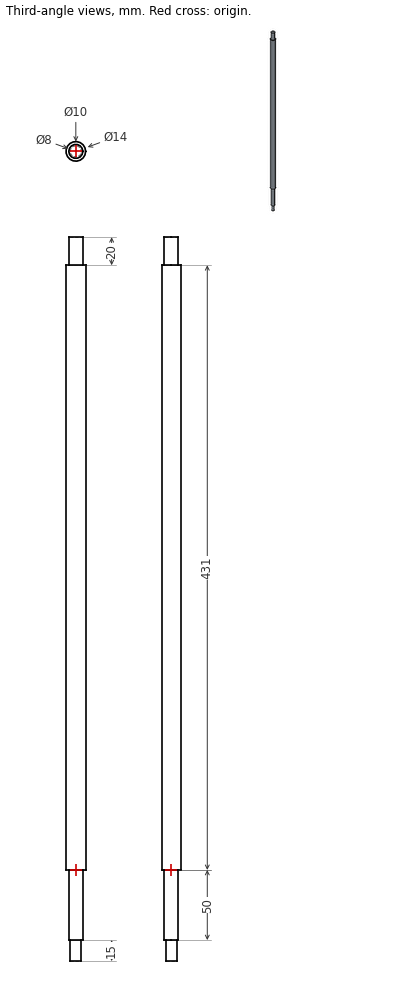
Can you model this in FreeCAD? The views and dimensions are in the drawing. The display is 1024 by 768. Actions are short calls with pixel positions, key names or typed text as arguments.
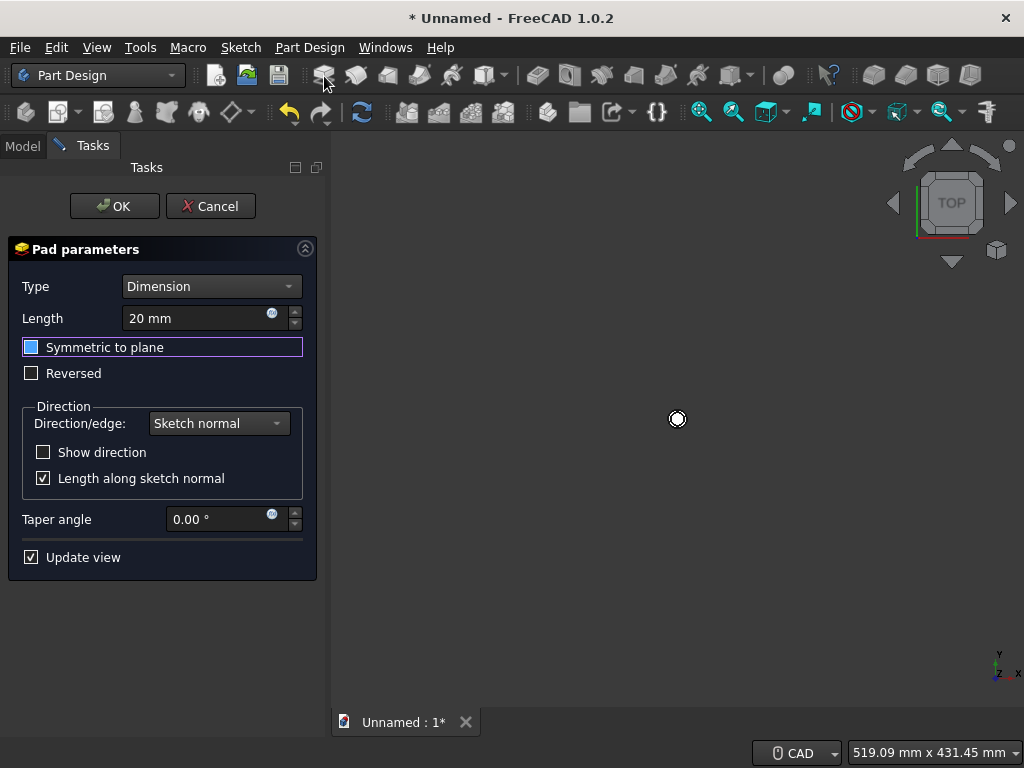
click(115, 206)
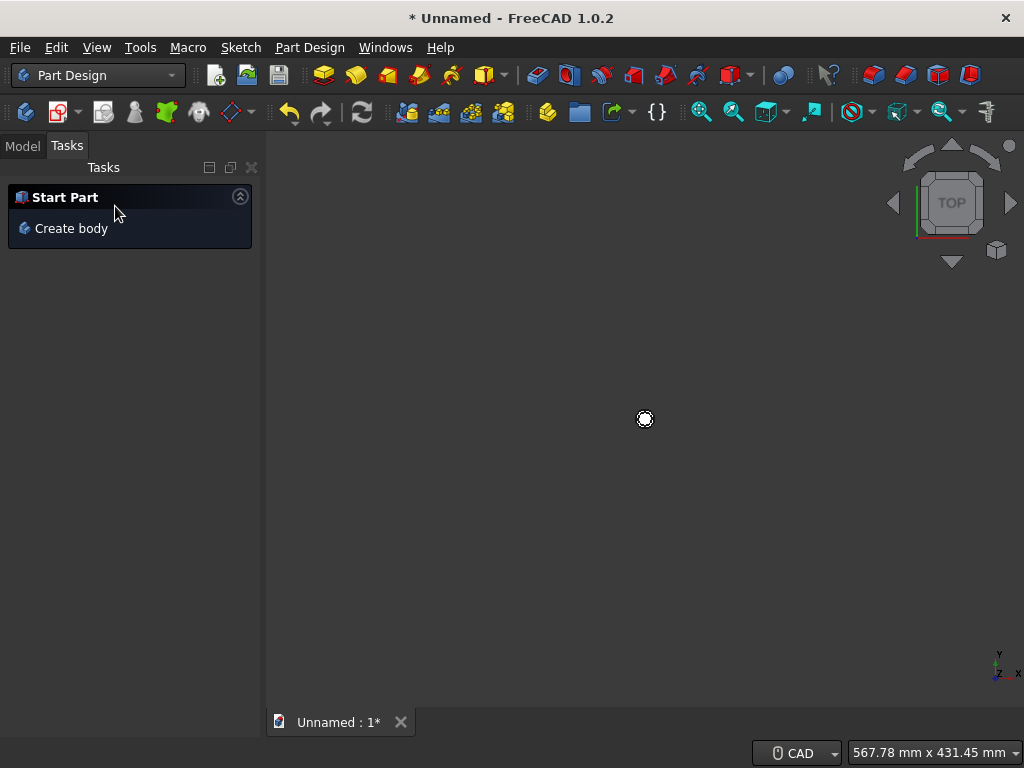
key(v)
key(f)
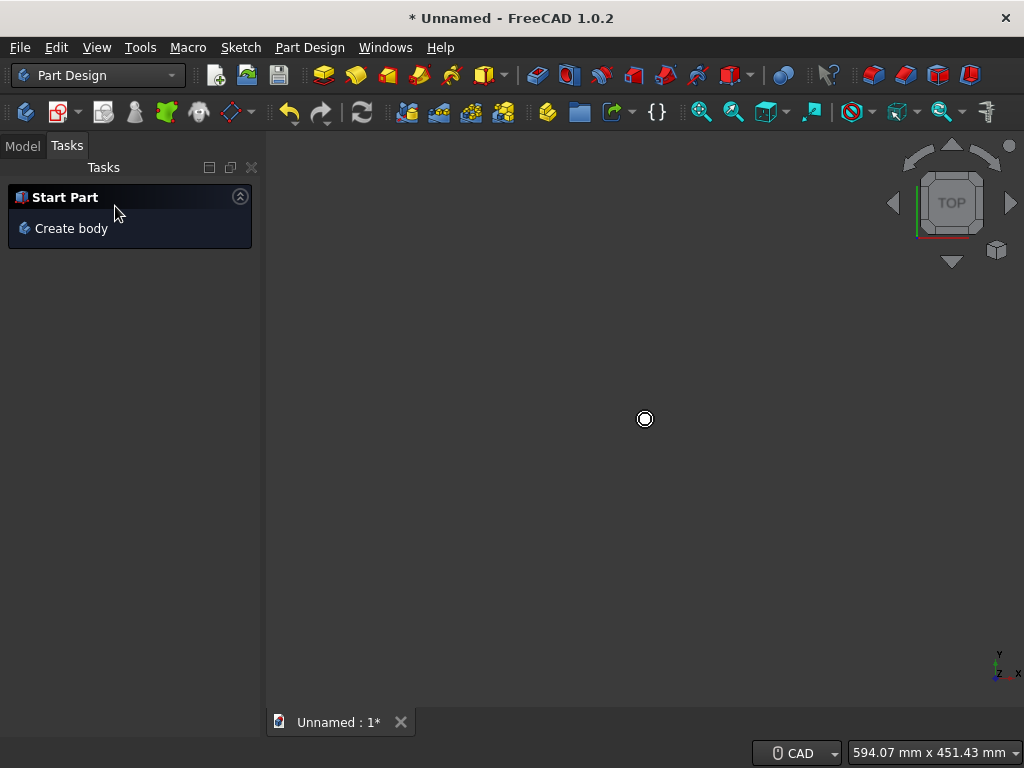
click(23, 145)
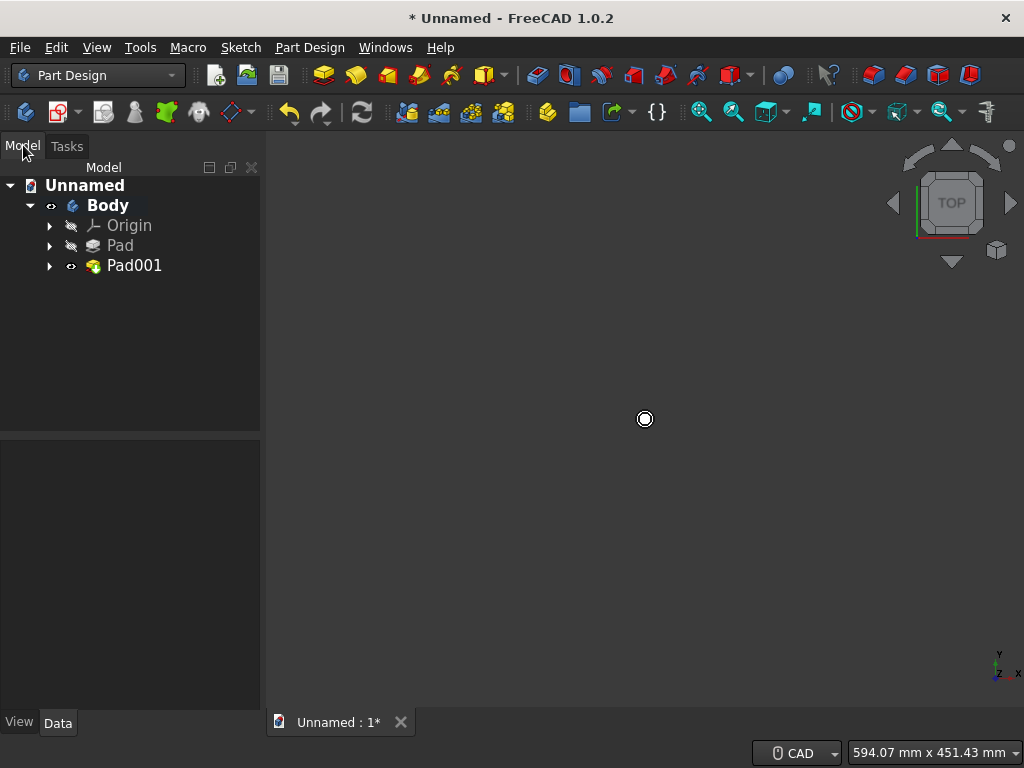
click(50, 226)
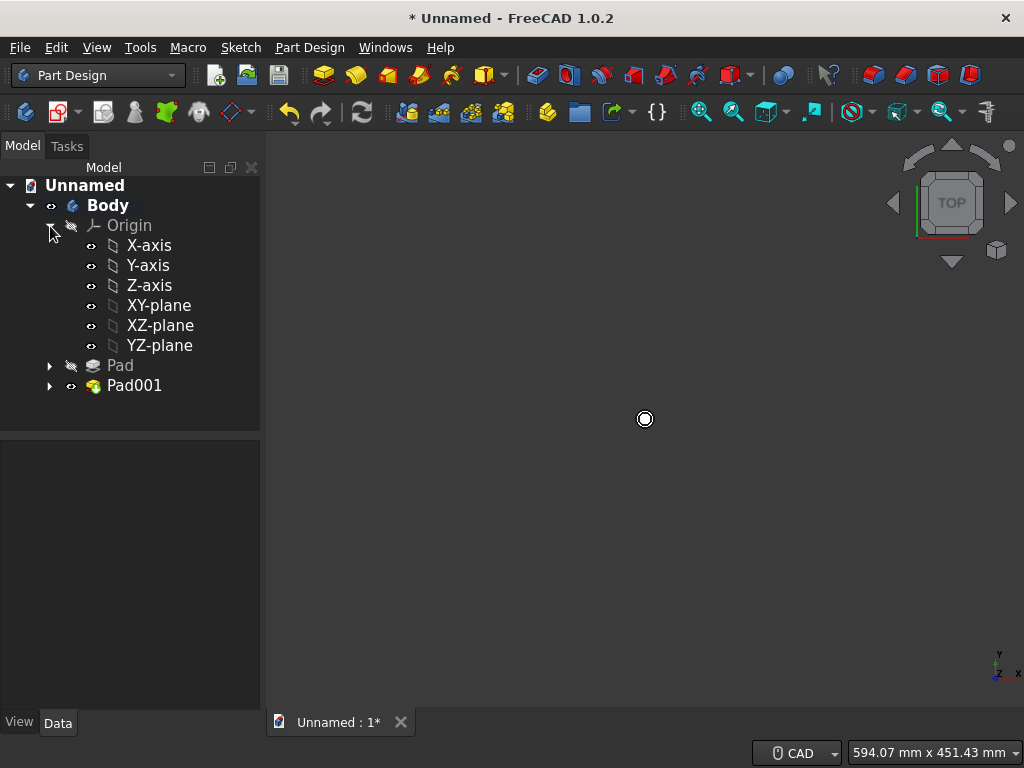
click(136, 306)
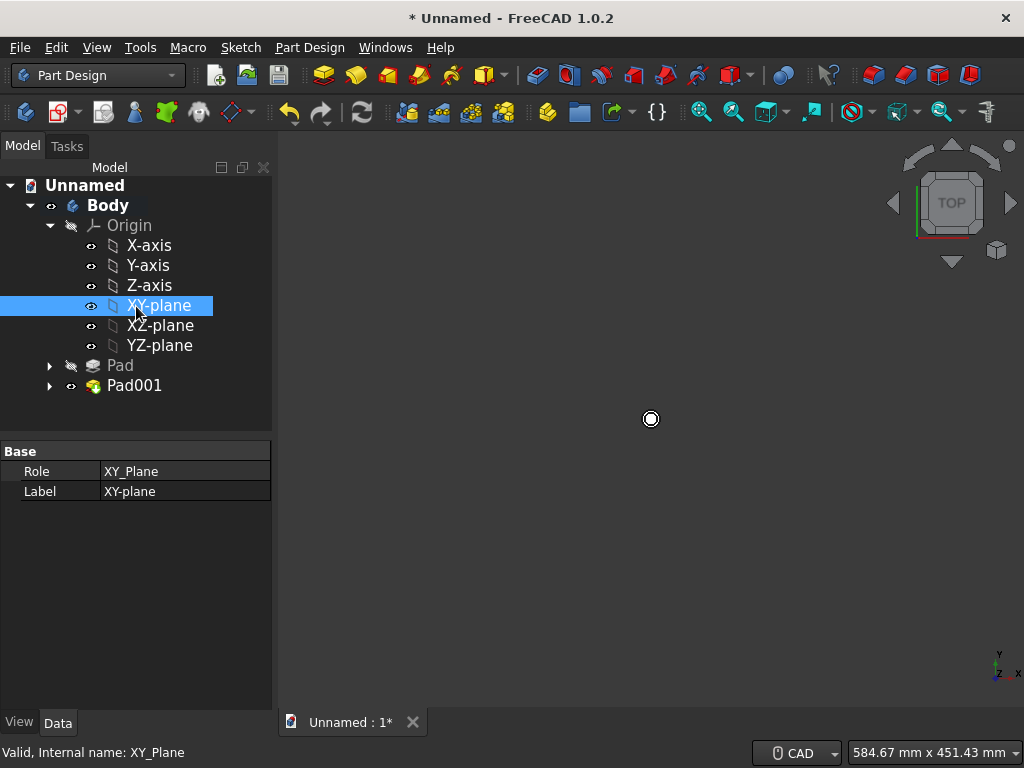
click(232, 112)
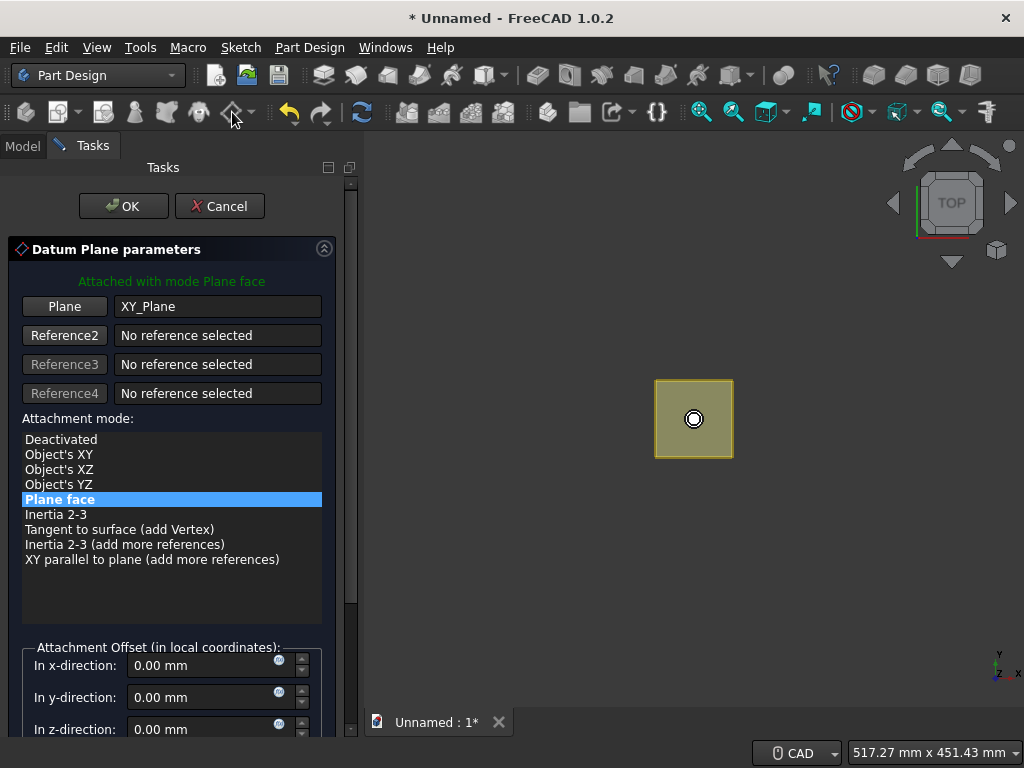
scroll(351, 456, down, 2)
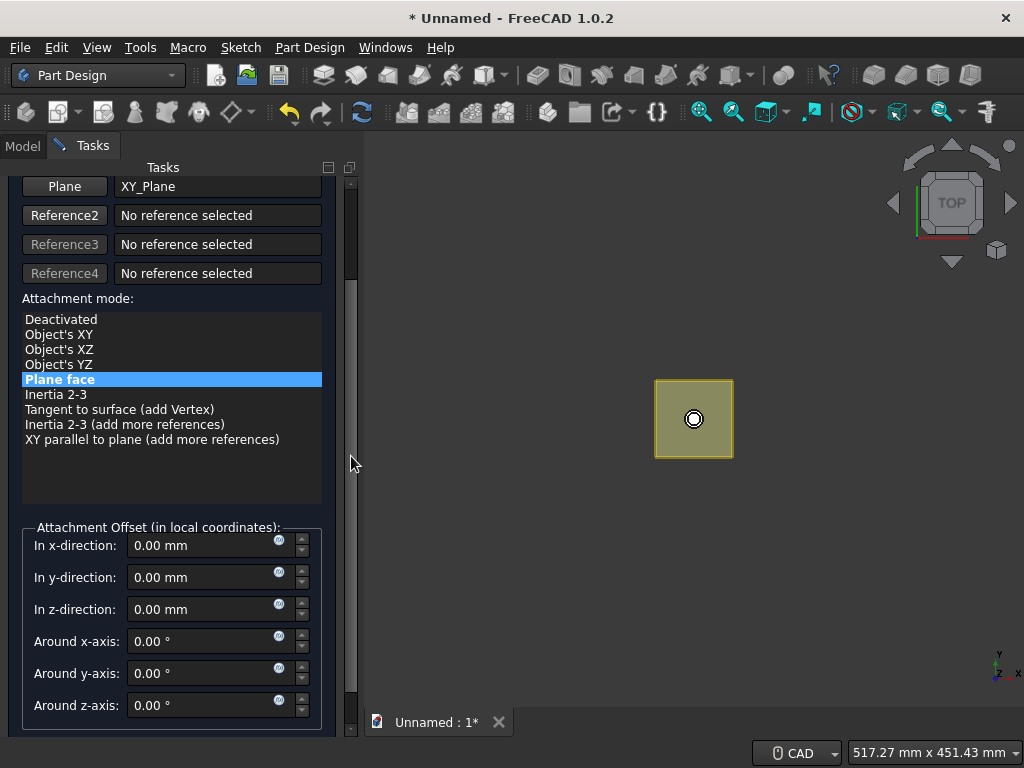
triple_click(210, 609)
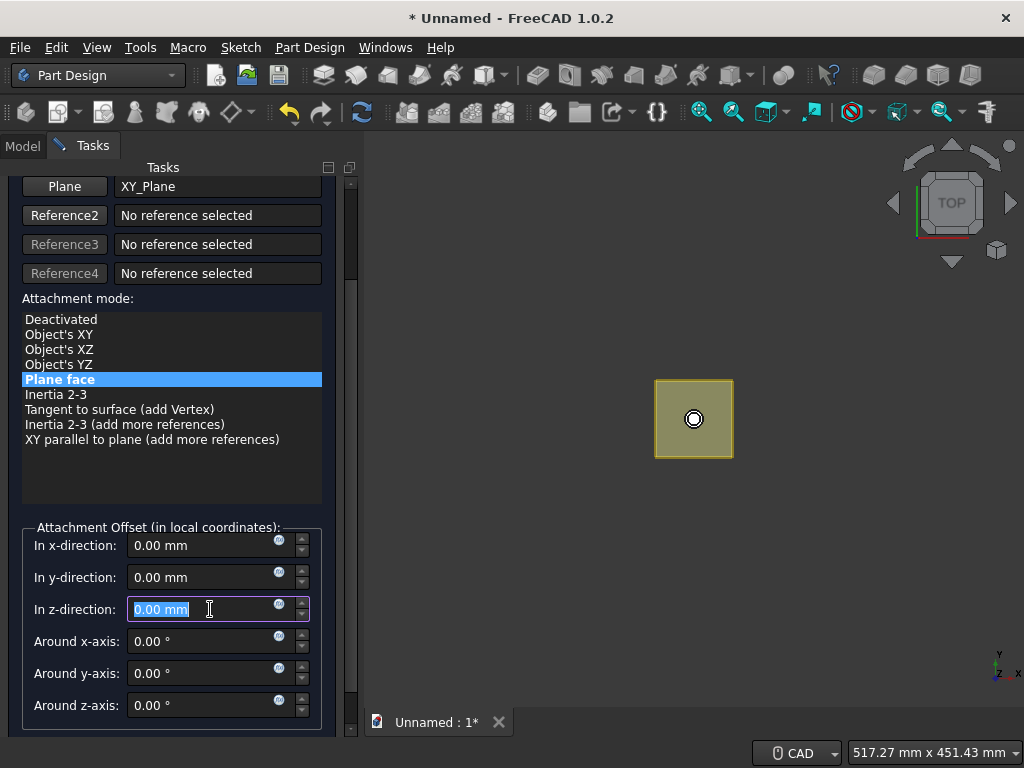
text(-50)
key(Tab)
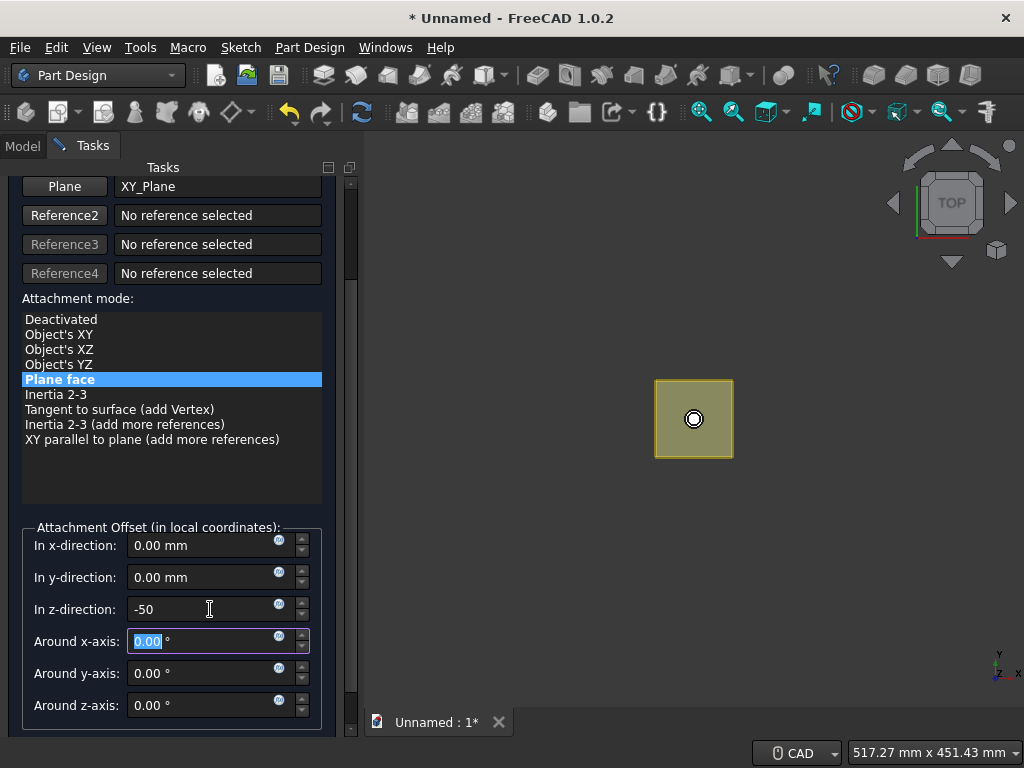
scroll(351, 456, up, 3)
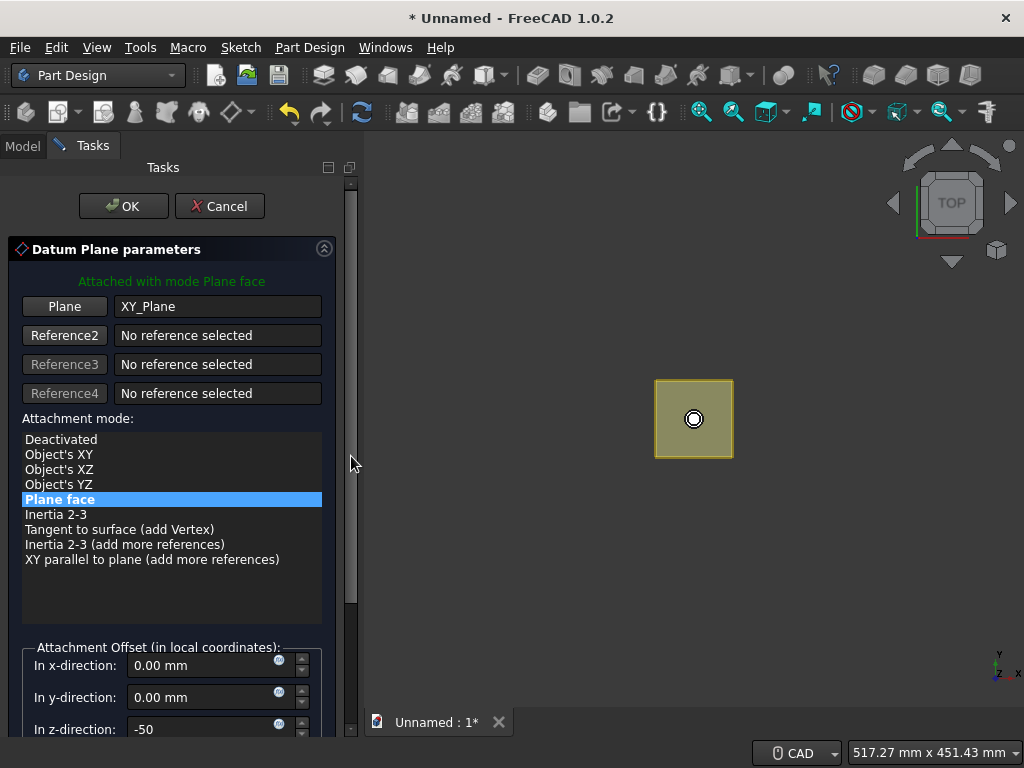
click(124, 206)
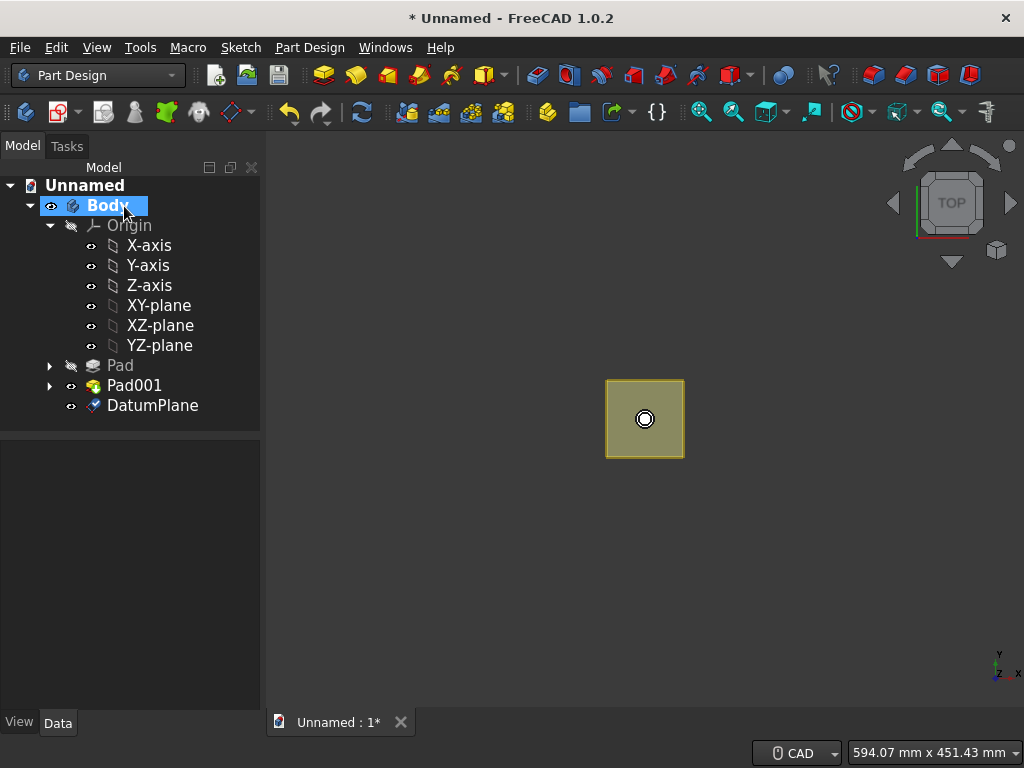
click(116, 406)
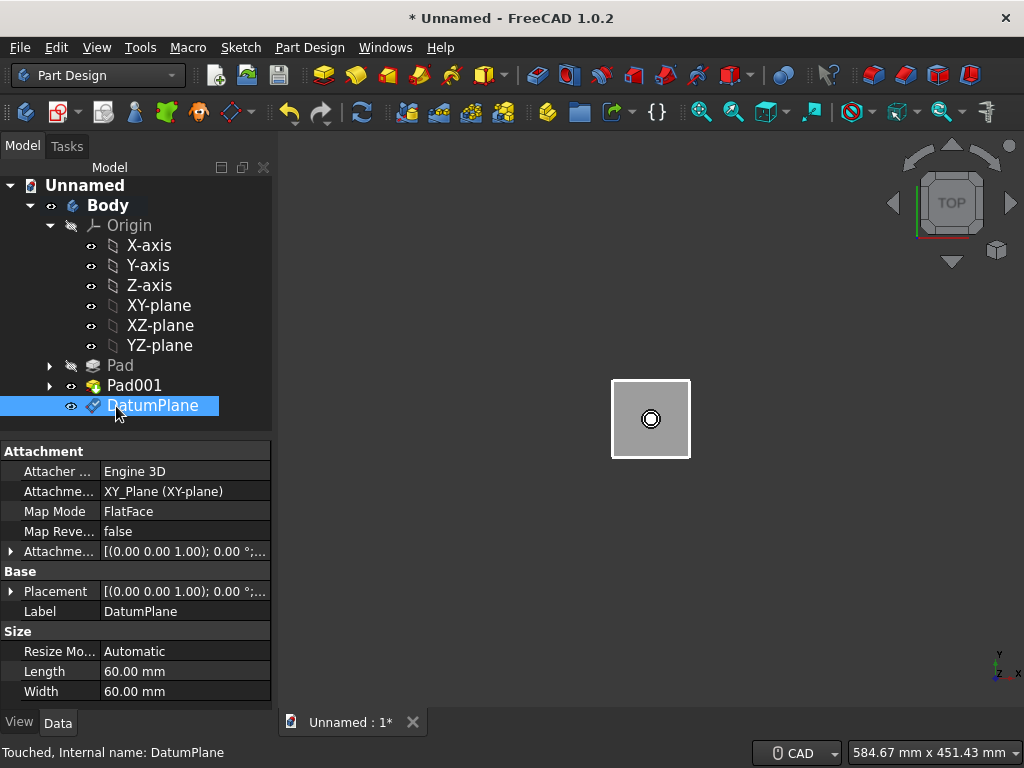
click(58, 112)